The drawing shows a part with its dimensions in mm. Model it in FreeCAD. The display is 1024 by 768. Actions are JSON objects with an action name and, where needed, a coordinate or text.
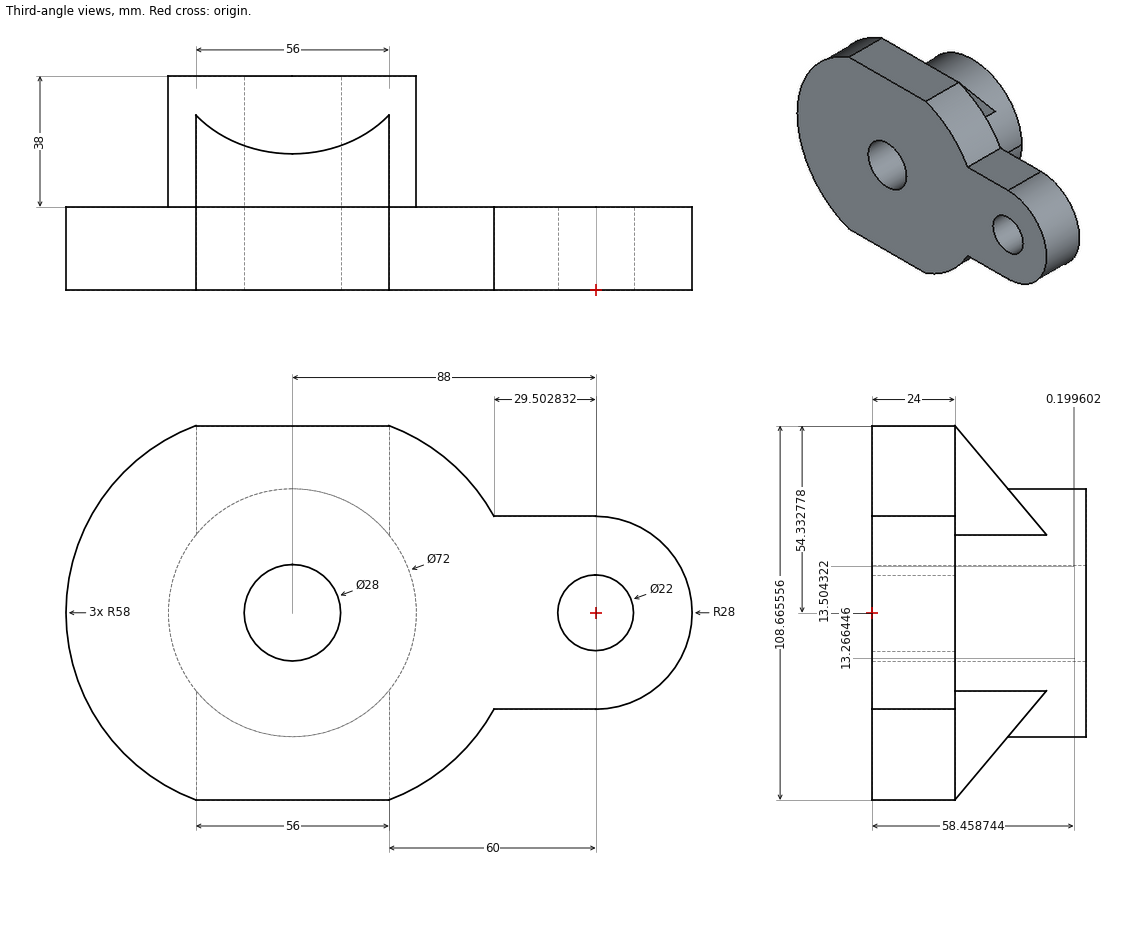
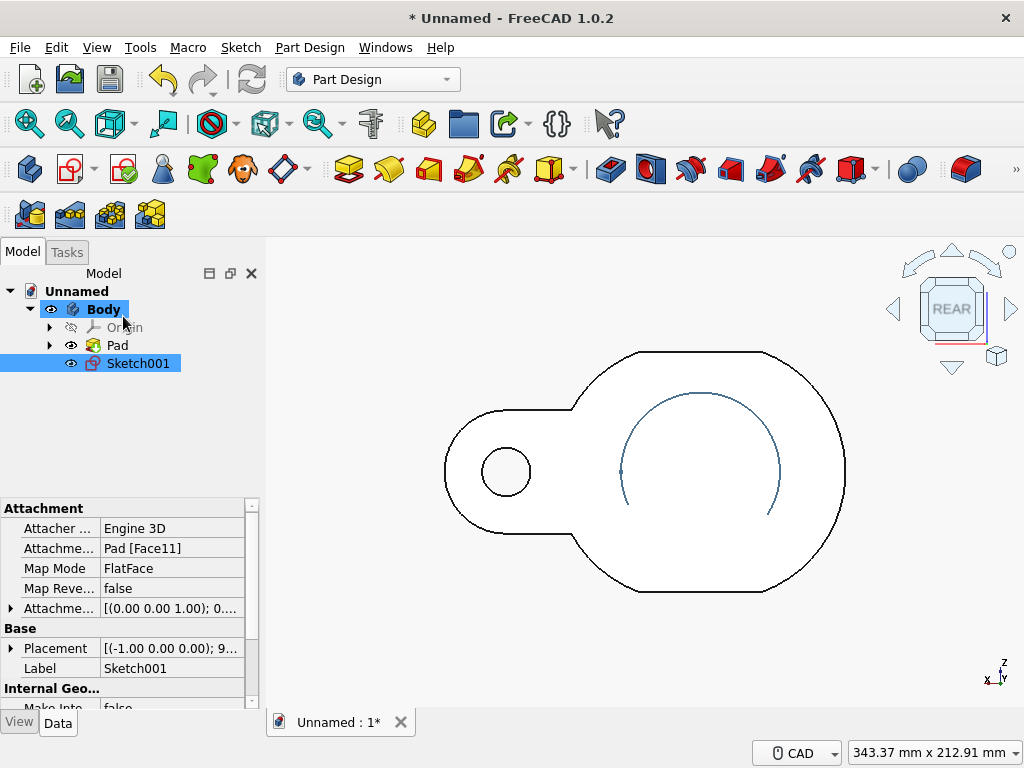
{"action": "left_click", "coordinate": [350, 170]}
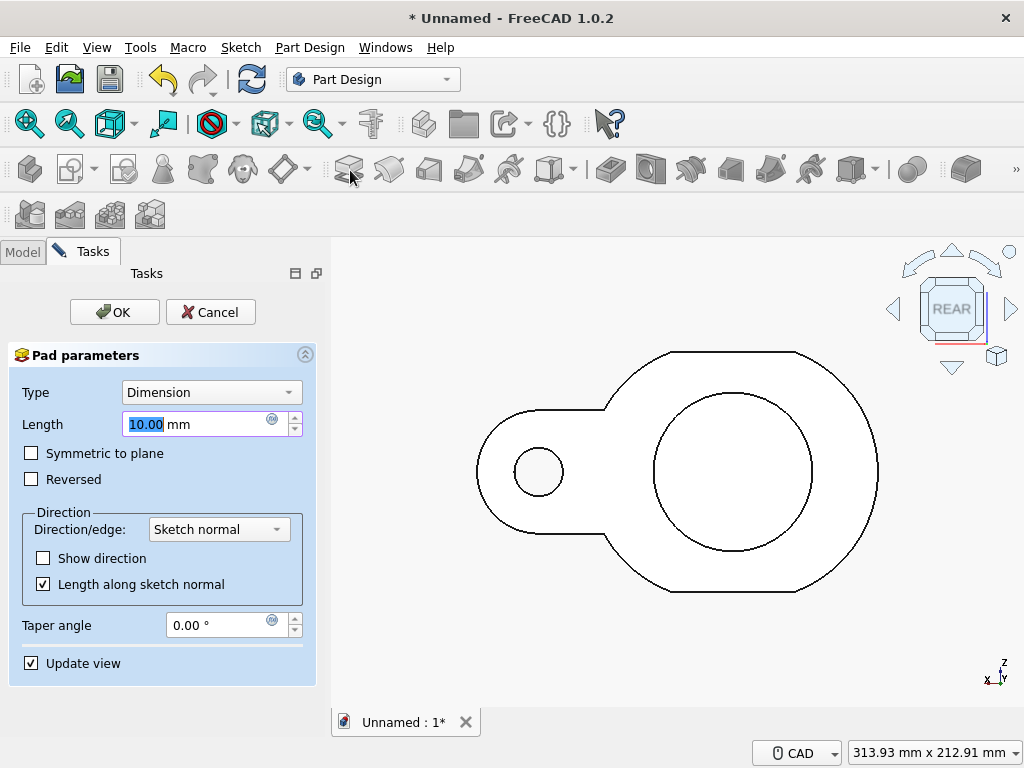
{"action": "type", "text": "38"}
{"action": "key", "text": "Tab"}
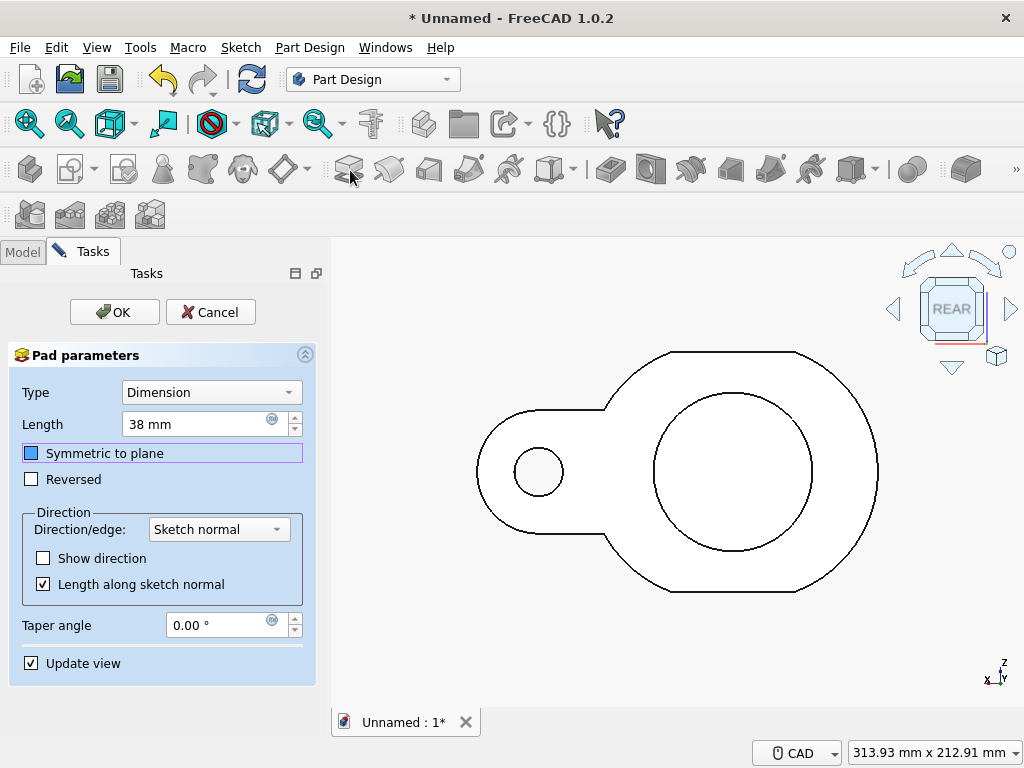
{"action": "left_click", "coordinate": [115, 312]}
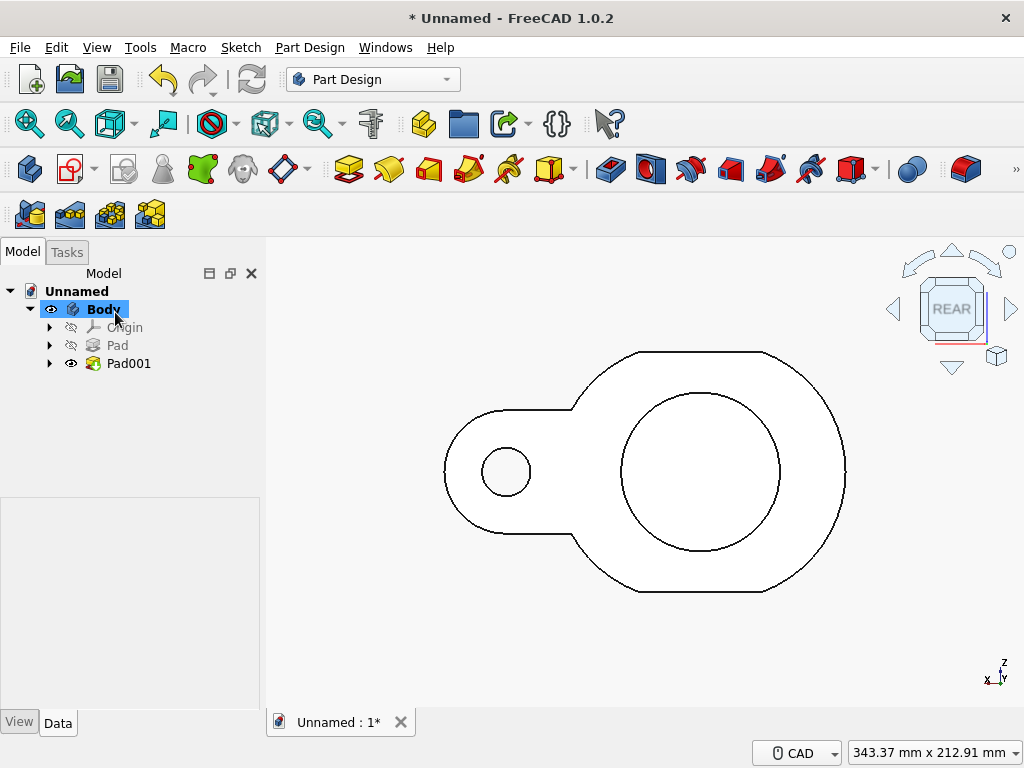
{"action": "left_click", "coordinate": [50, 327]}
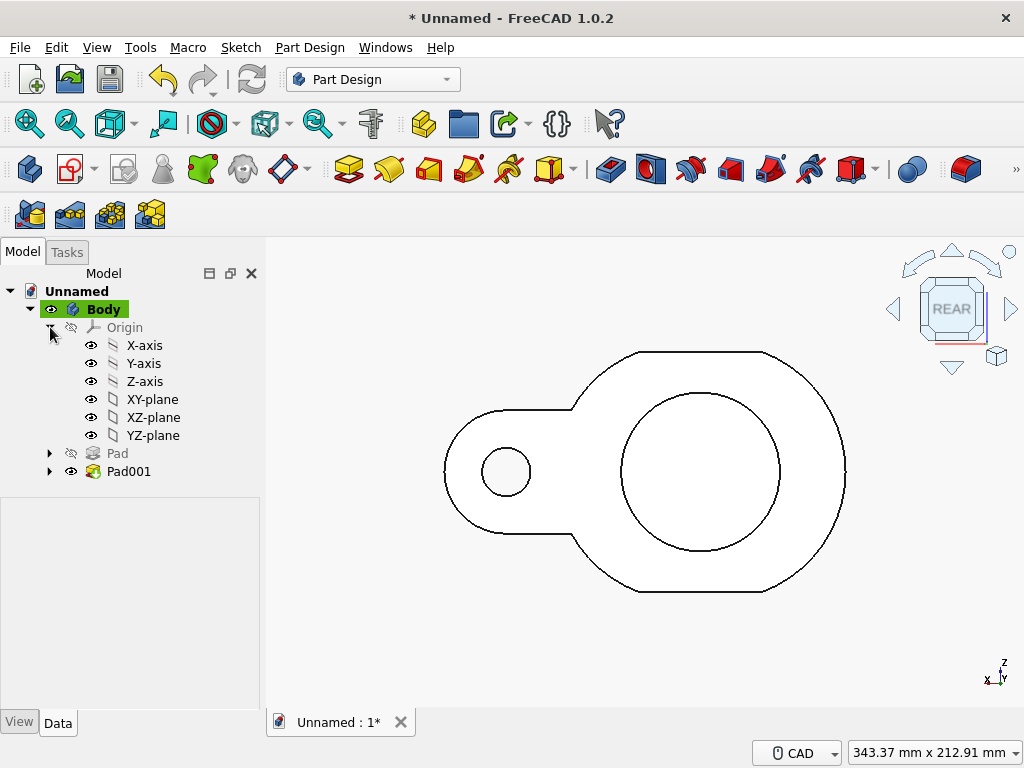
{"action": "left_click", "coordinate": [136, 435]}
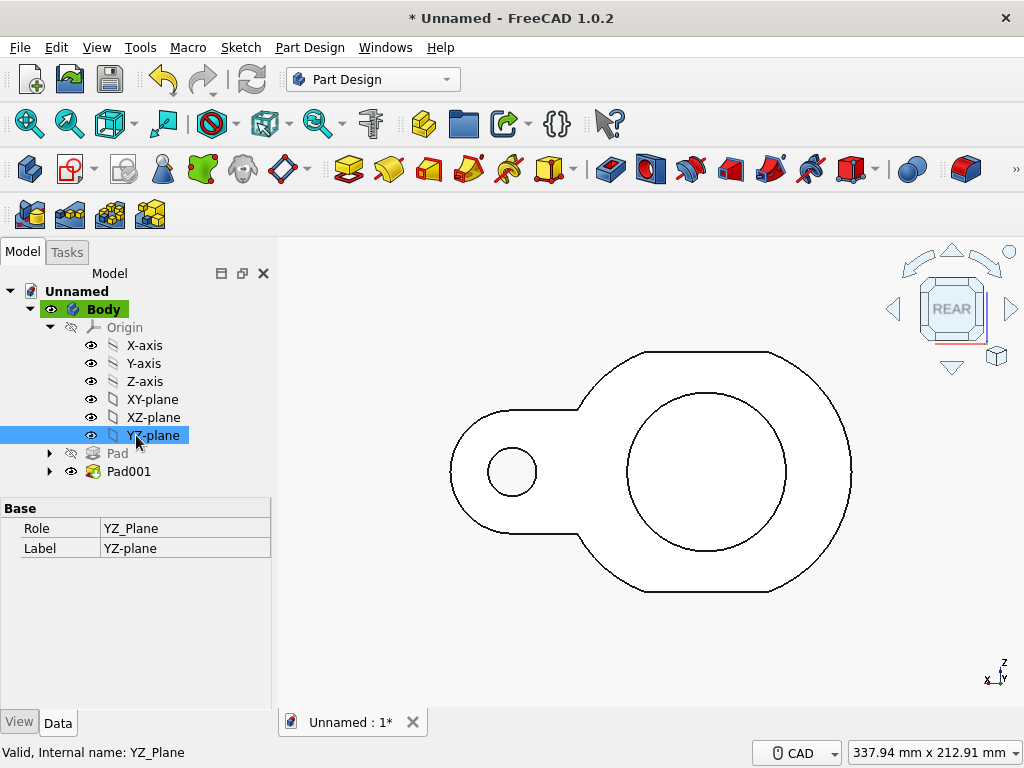
{"action": "left_click", "coordinate": [284, 170]}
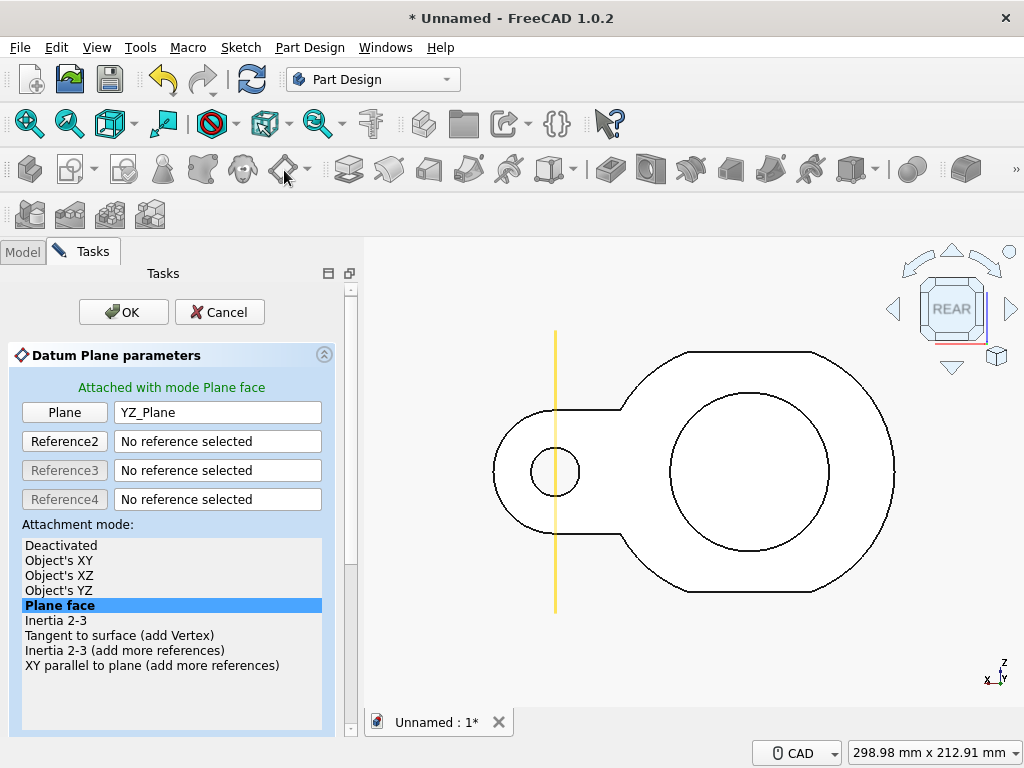
{"action": "scroll", "coordinate": [351, 510], "scroll_direction": "down", "scroll_amount": 3}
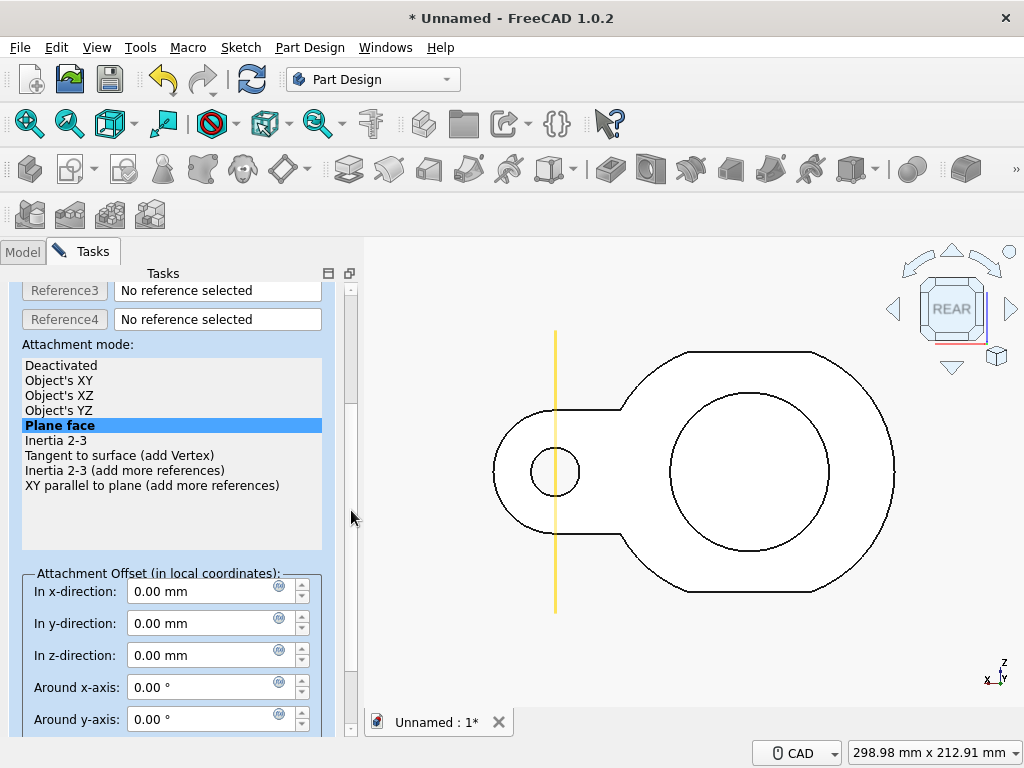
{"action": "triple_click", "coordinate": [210, 655]}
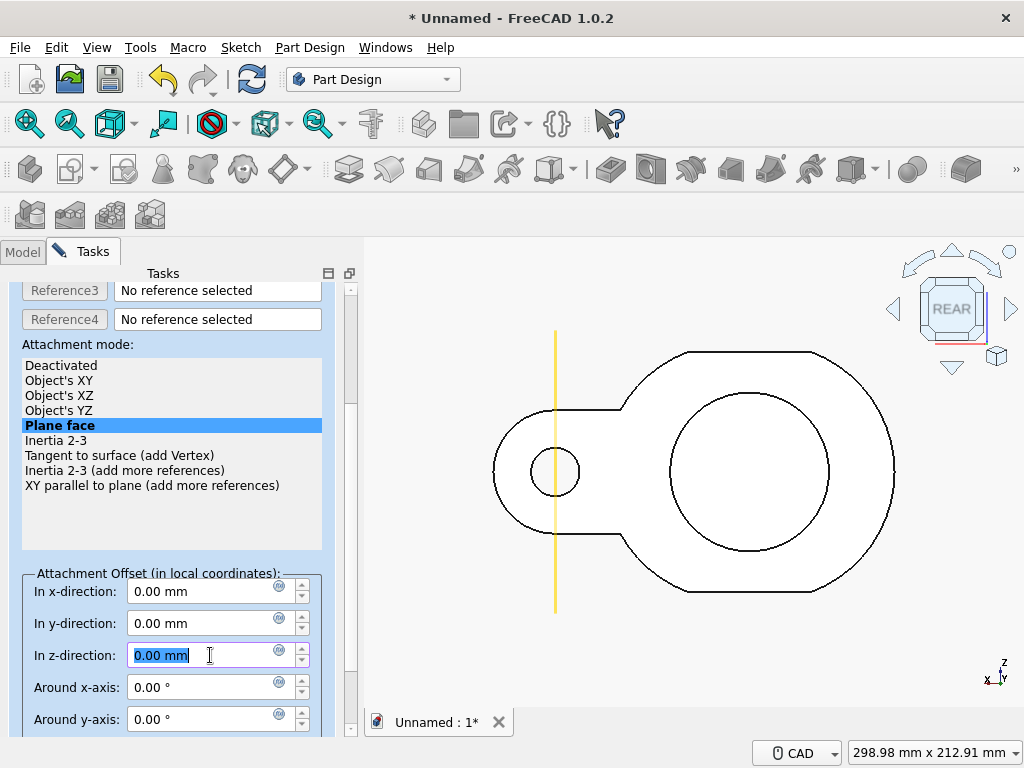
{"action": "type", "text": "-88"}
{"action": "key", "text": "Tab"}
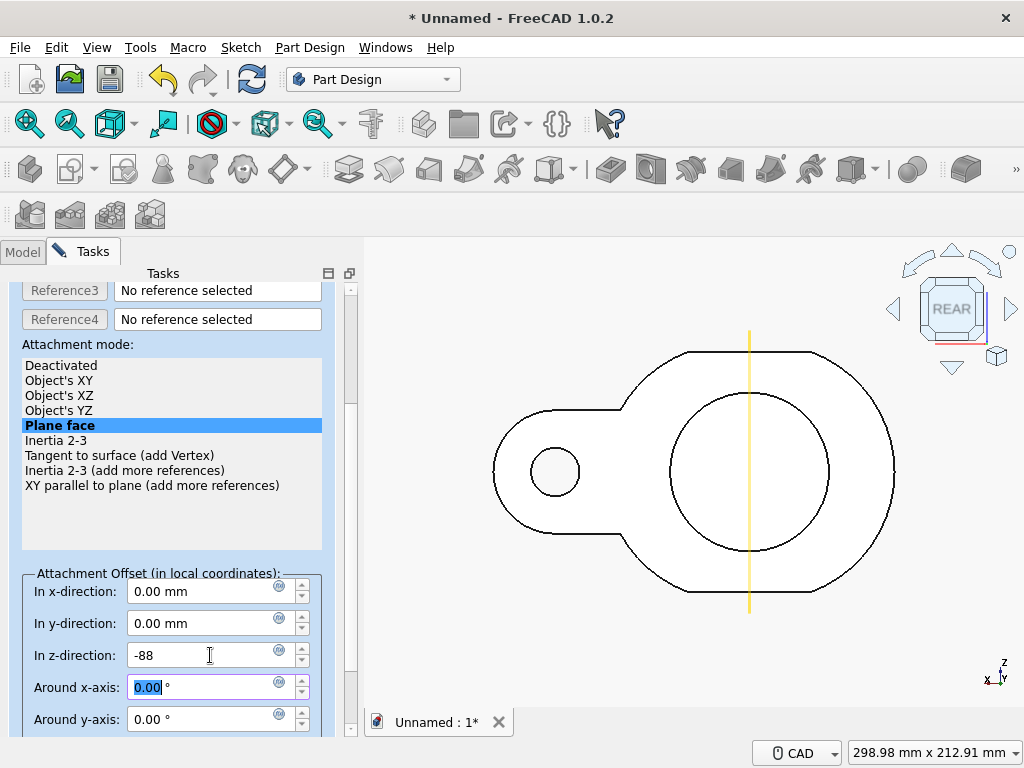
{"action": "scroll", "coordinate": [351, 510], "scroll_direction": "up", "scroll_amount": 4}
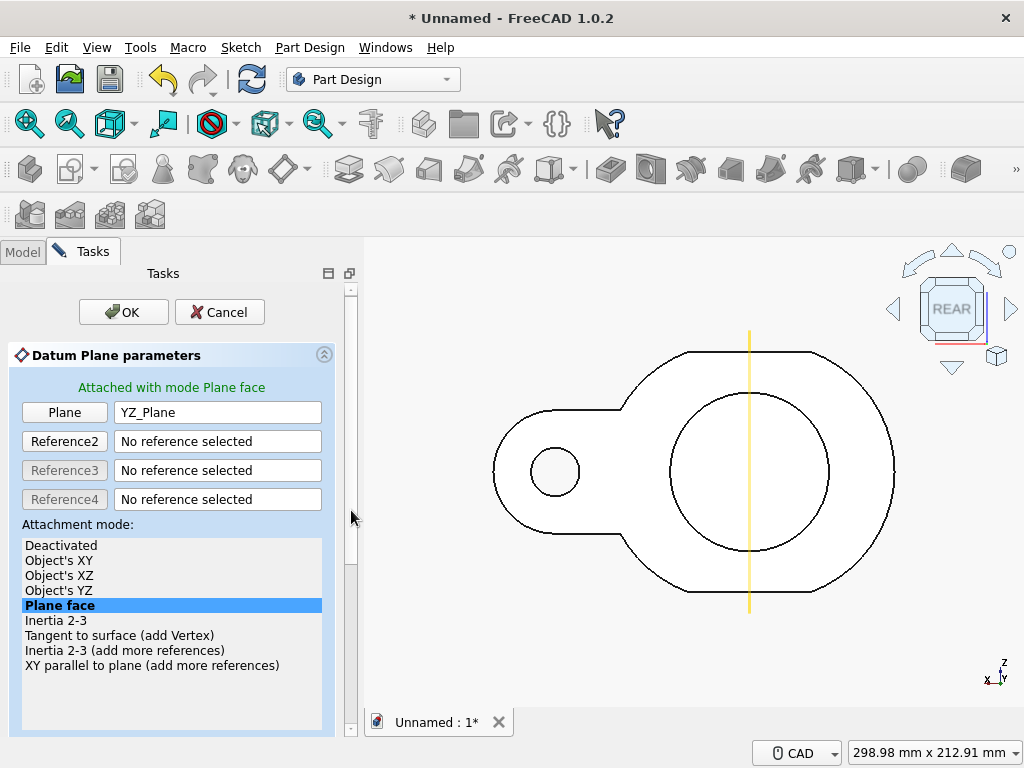
{"action": "left_click", "coordinate": [124, 312]}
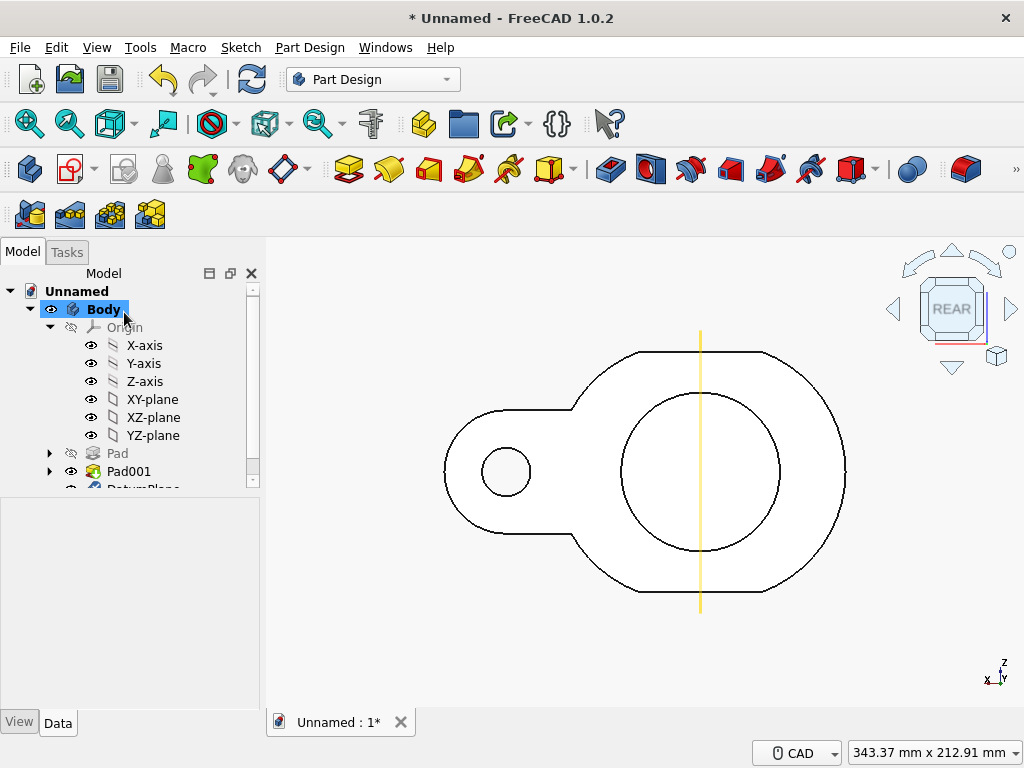
{"action": "scroll", "coordinate": [100, 377], "scroll_direction": "down", "scroll_amount": 3}